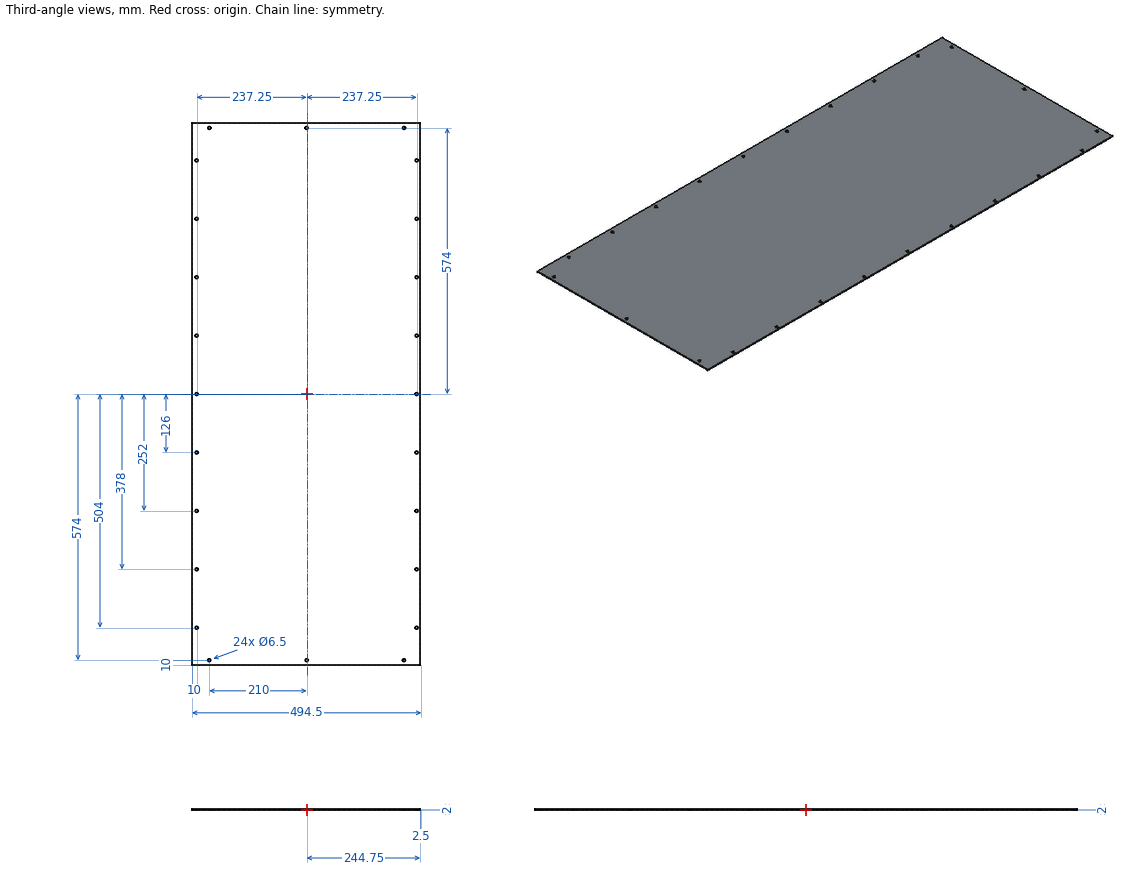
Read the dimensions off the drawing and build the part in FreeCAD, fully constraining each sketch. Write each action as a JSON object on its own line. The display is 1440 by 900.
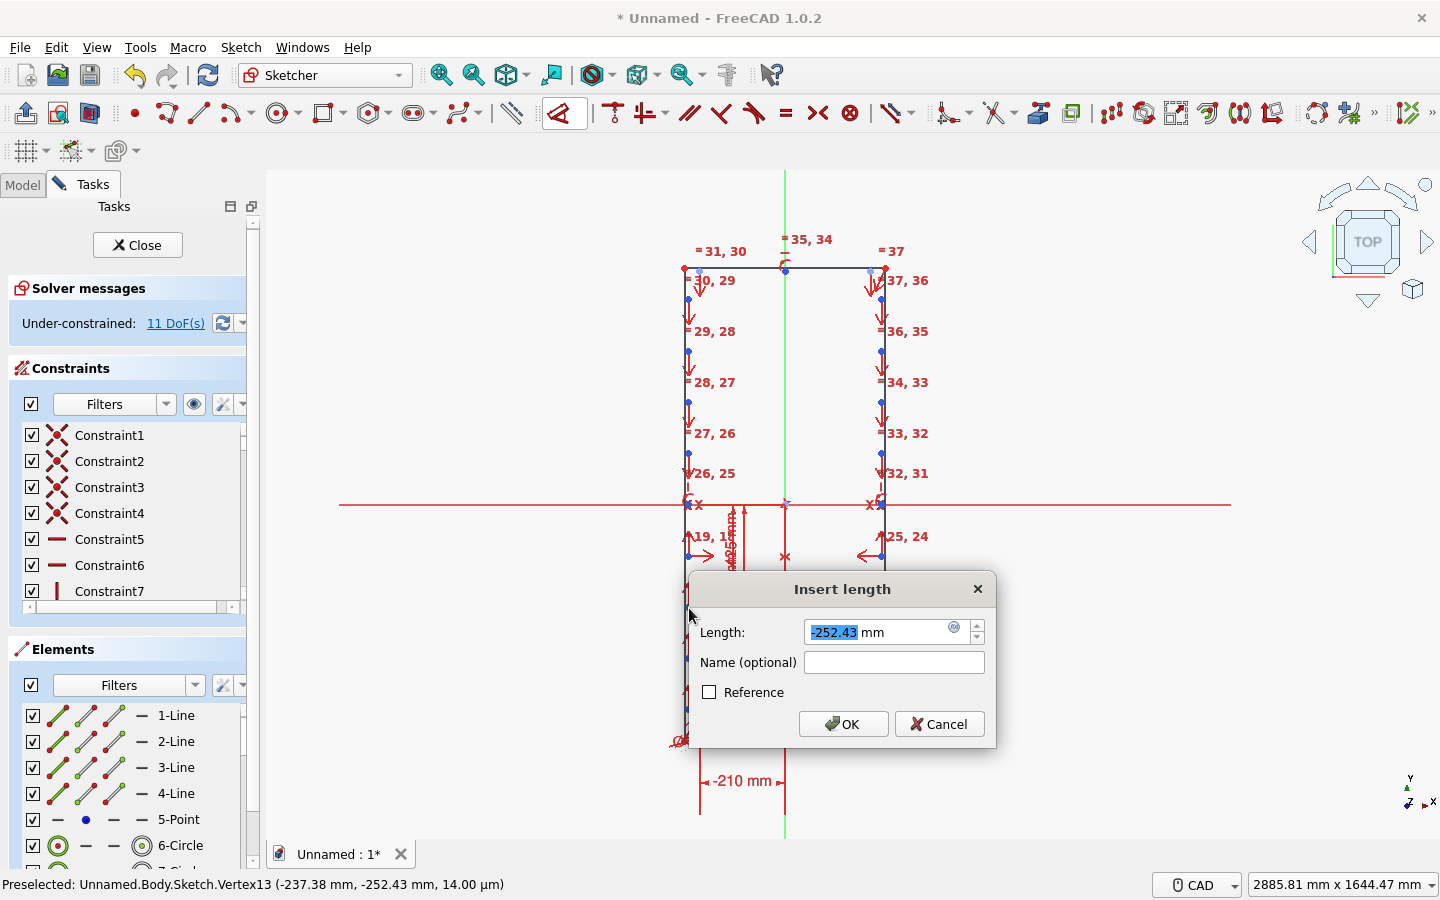
{"action": "type", "text": "-252"}
{"action": "key", "text": "Return"}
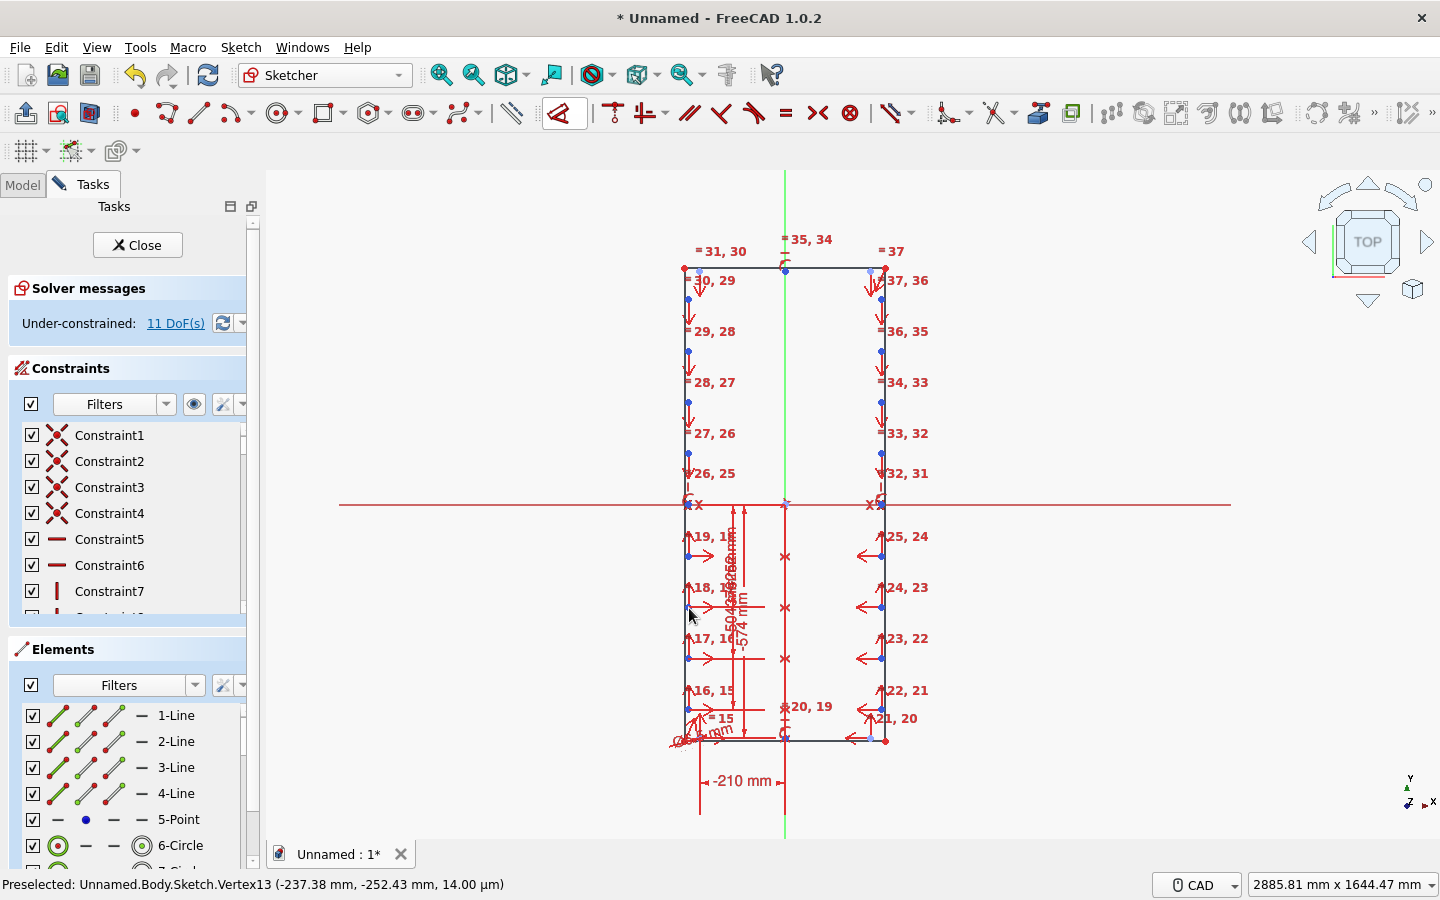
{"action": "left_click", "coordinate": [689, 556]}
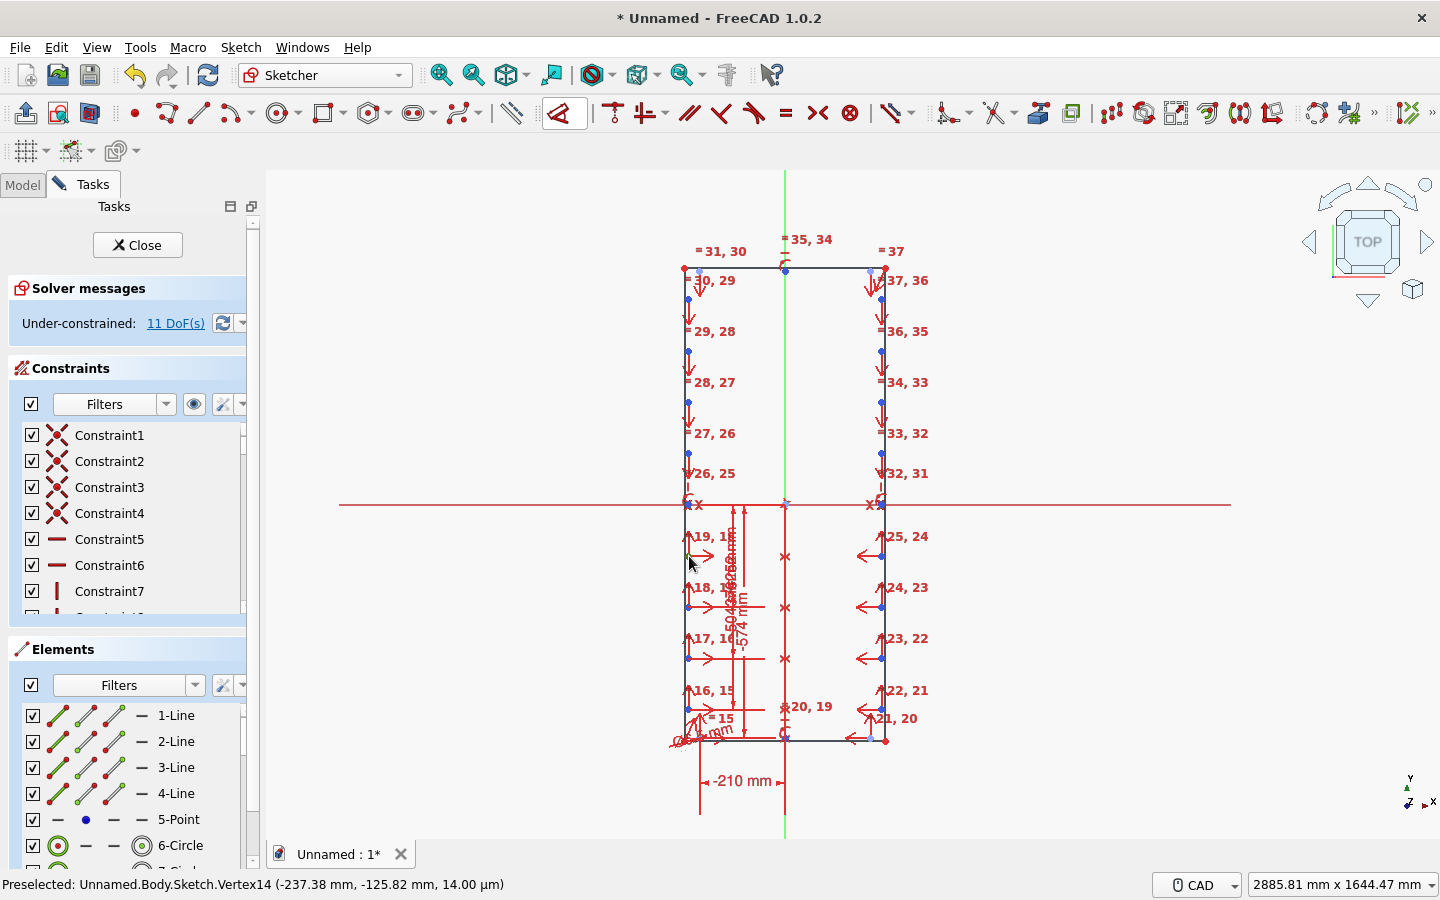
{"action": "key", "text": "i"}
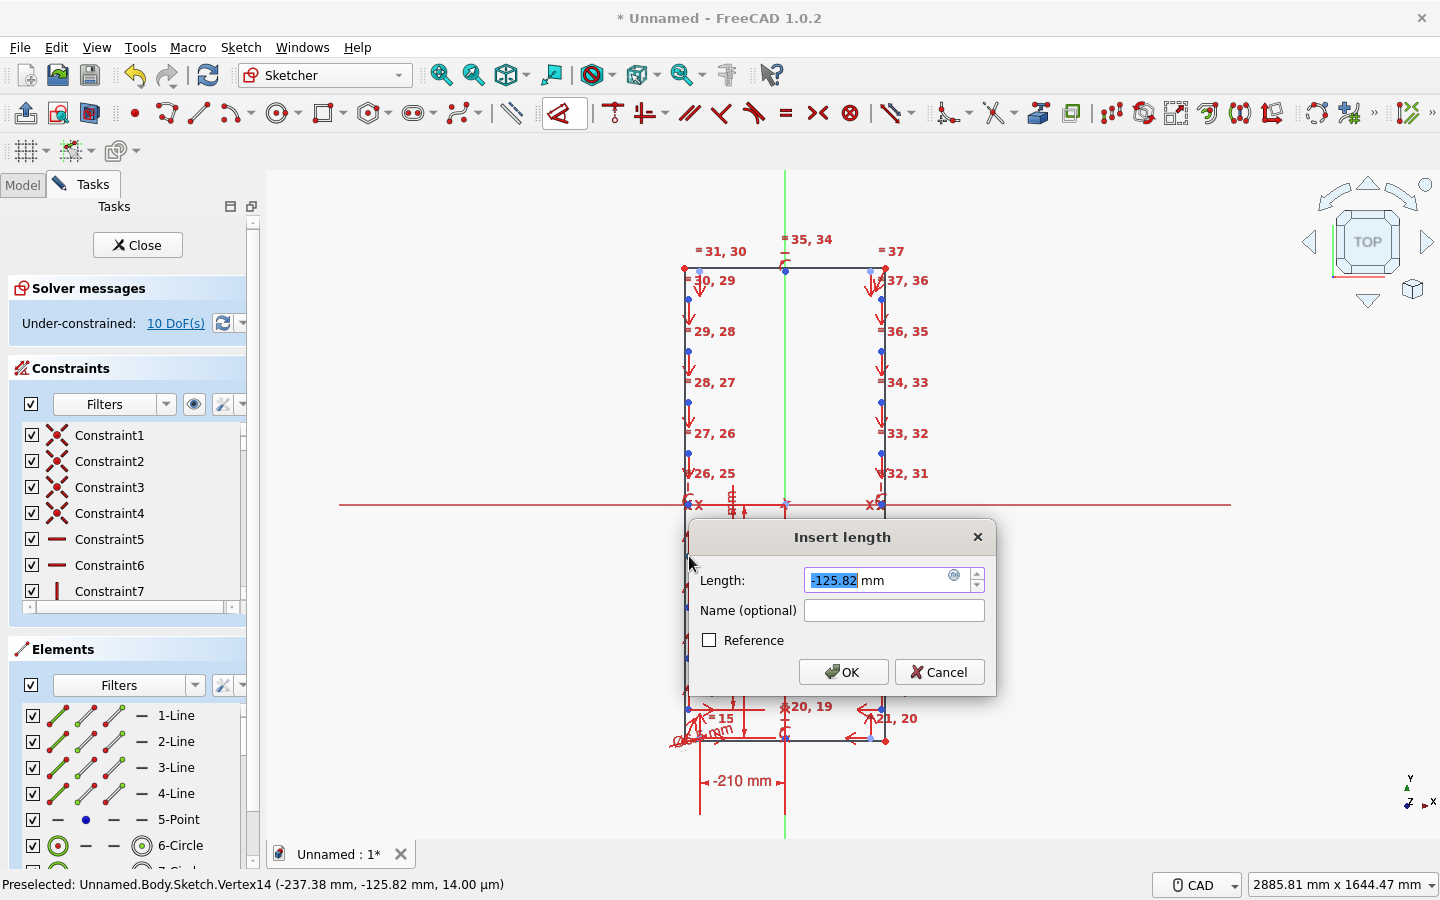
{"action": "type", "text": "-126"}
{"action": "key", "text": "Return"}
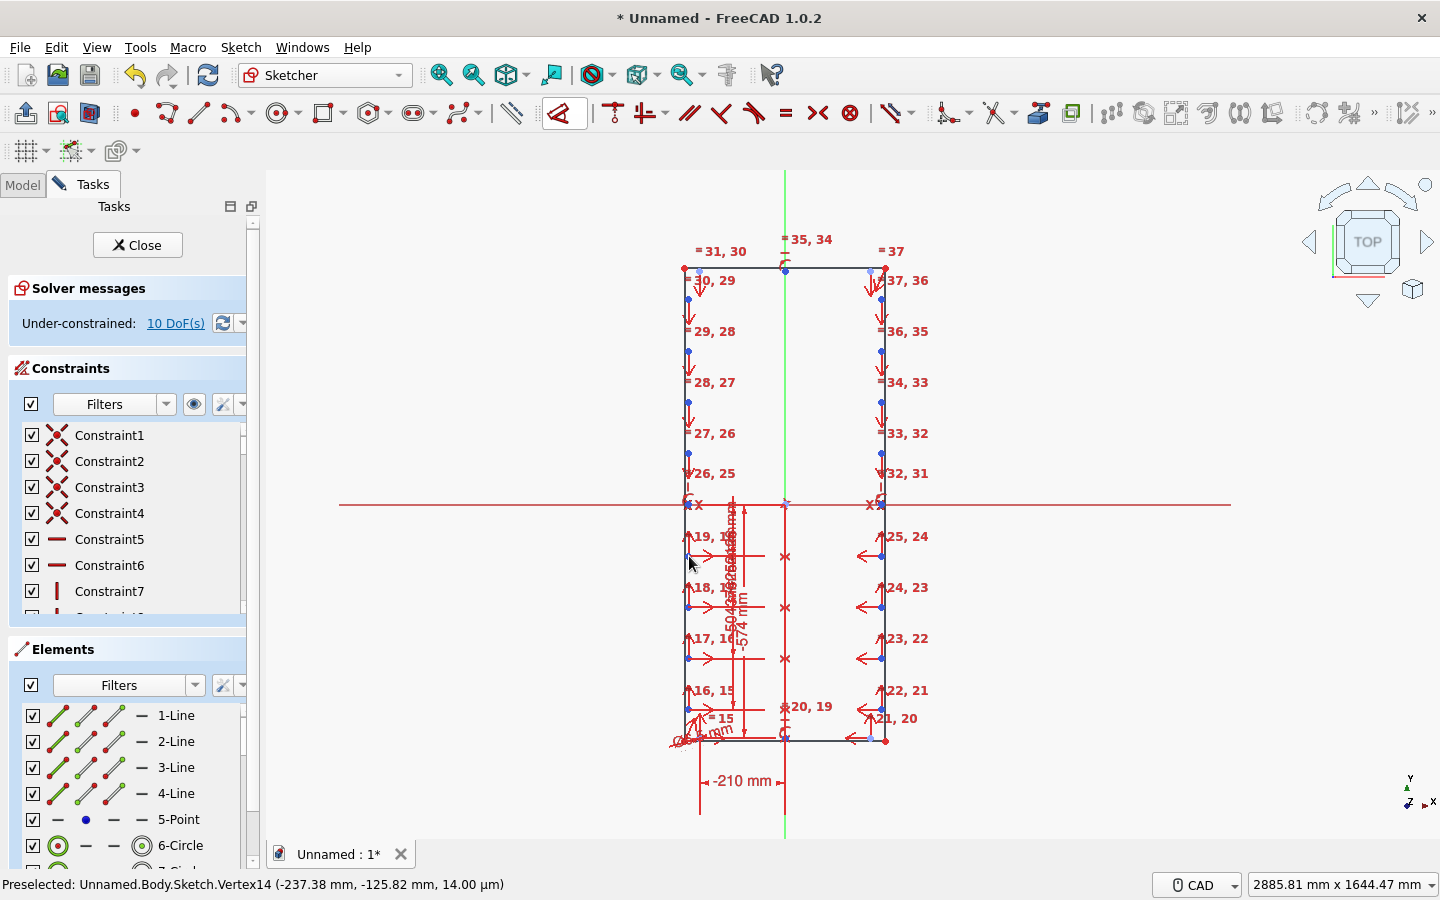
{"action": "left_click", "coordinate": [785, 739]}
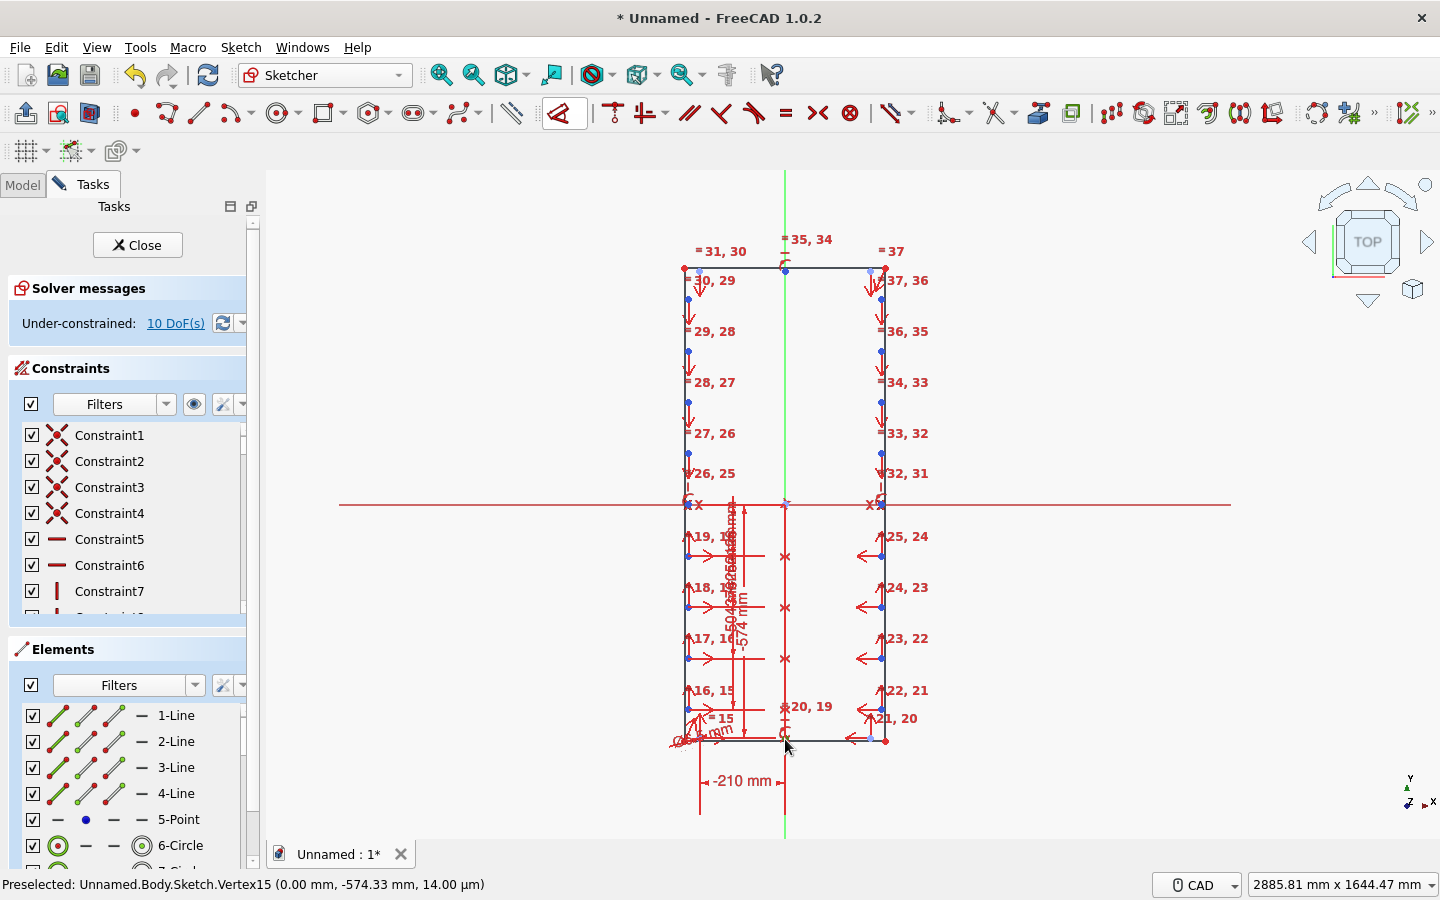
{"action": "left_click", "coordinate": [582, 114]}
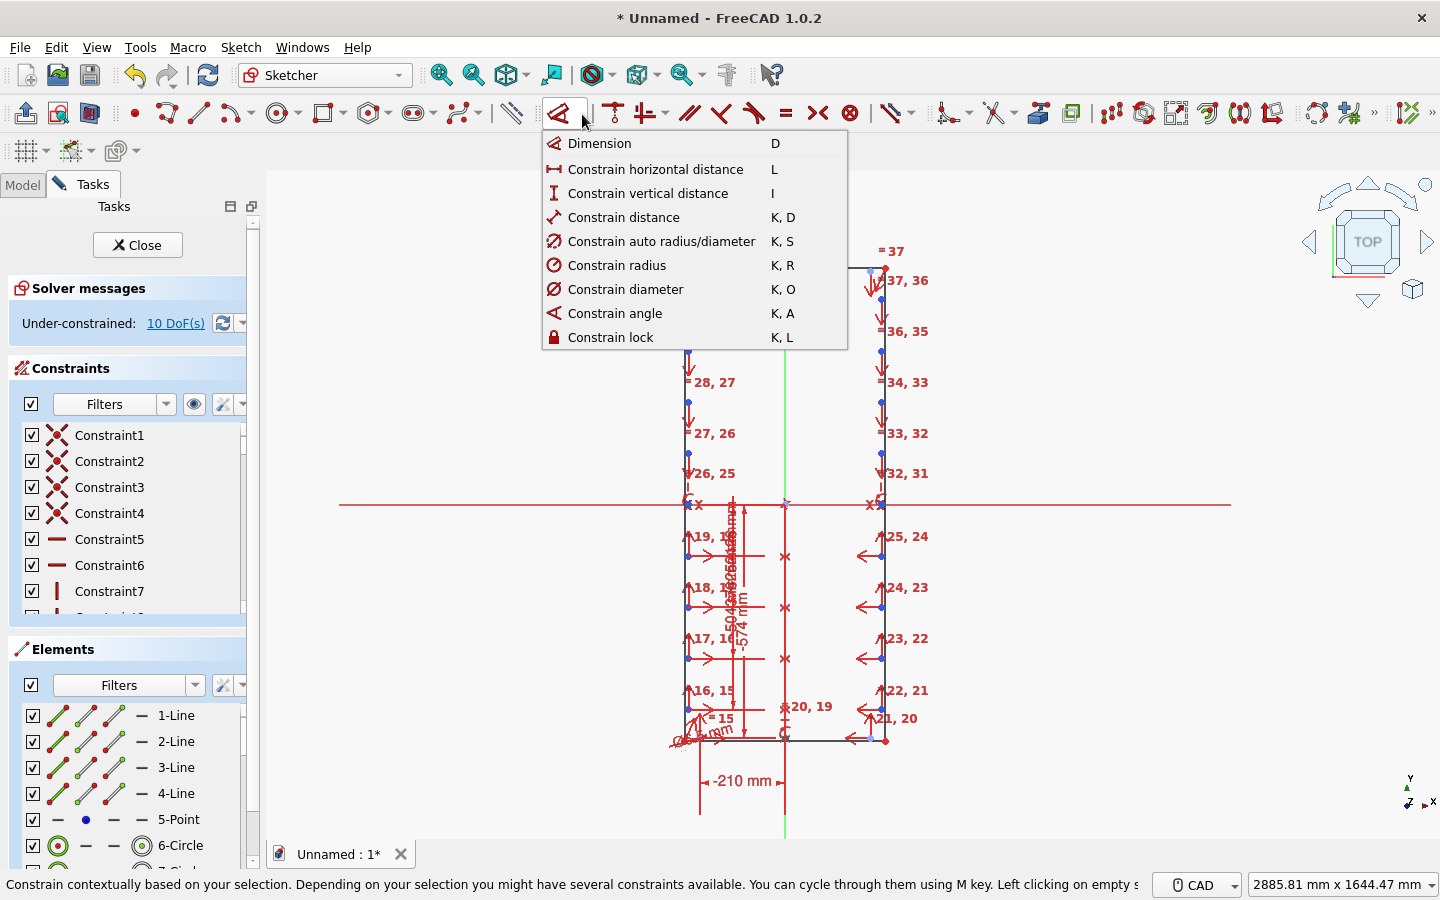
{"action": "left_click", "coordinate": [695, 193]}